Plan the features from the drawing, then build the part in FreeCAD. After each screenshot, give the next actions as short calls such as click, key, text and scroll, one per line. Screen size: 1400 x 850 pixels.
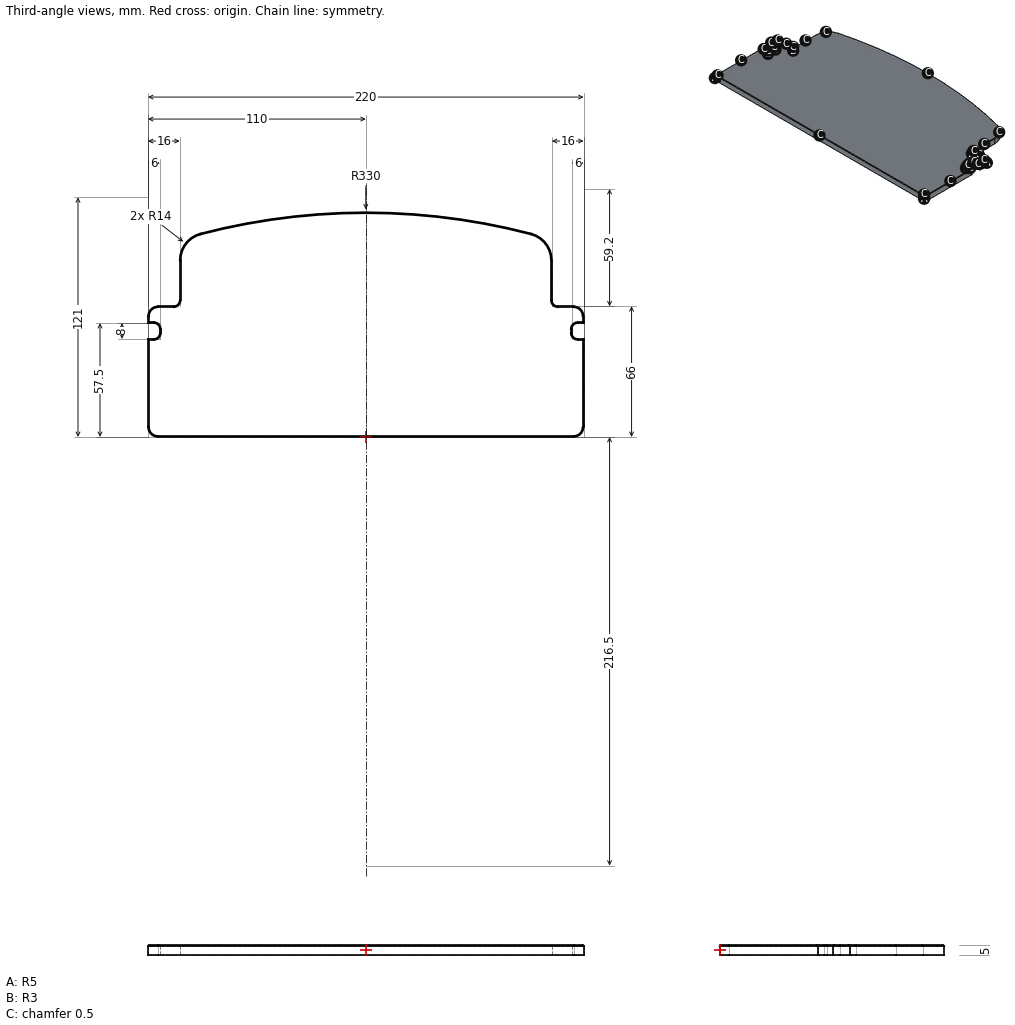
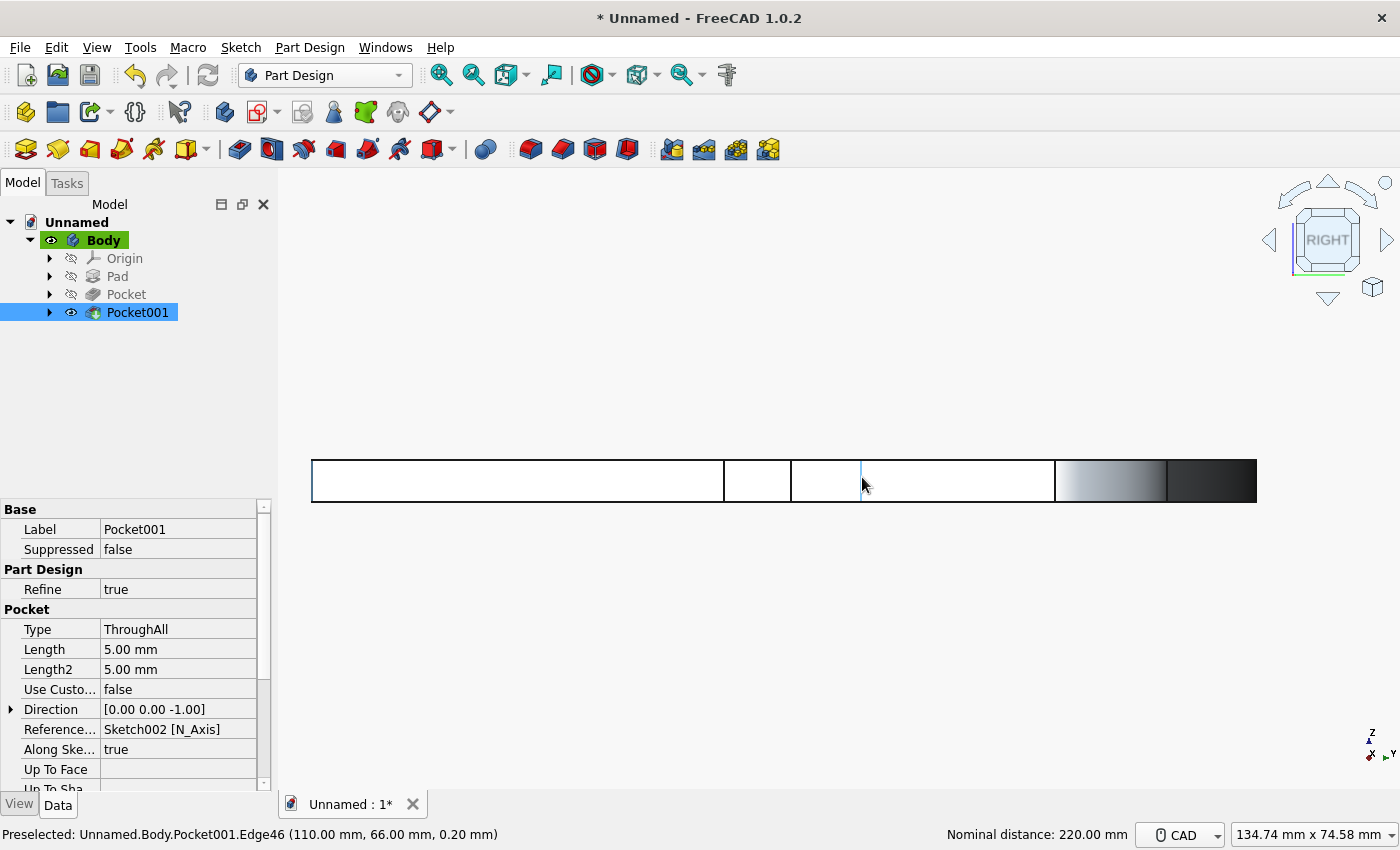
click(861, 480, ctrl)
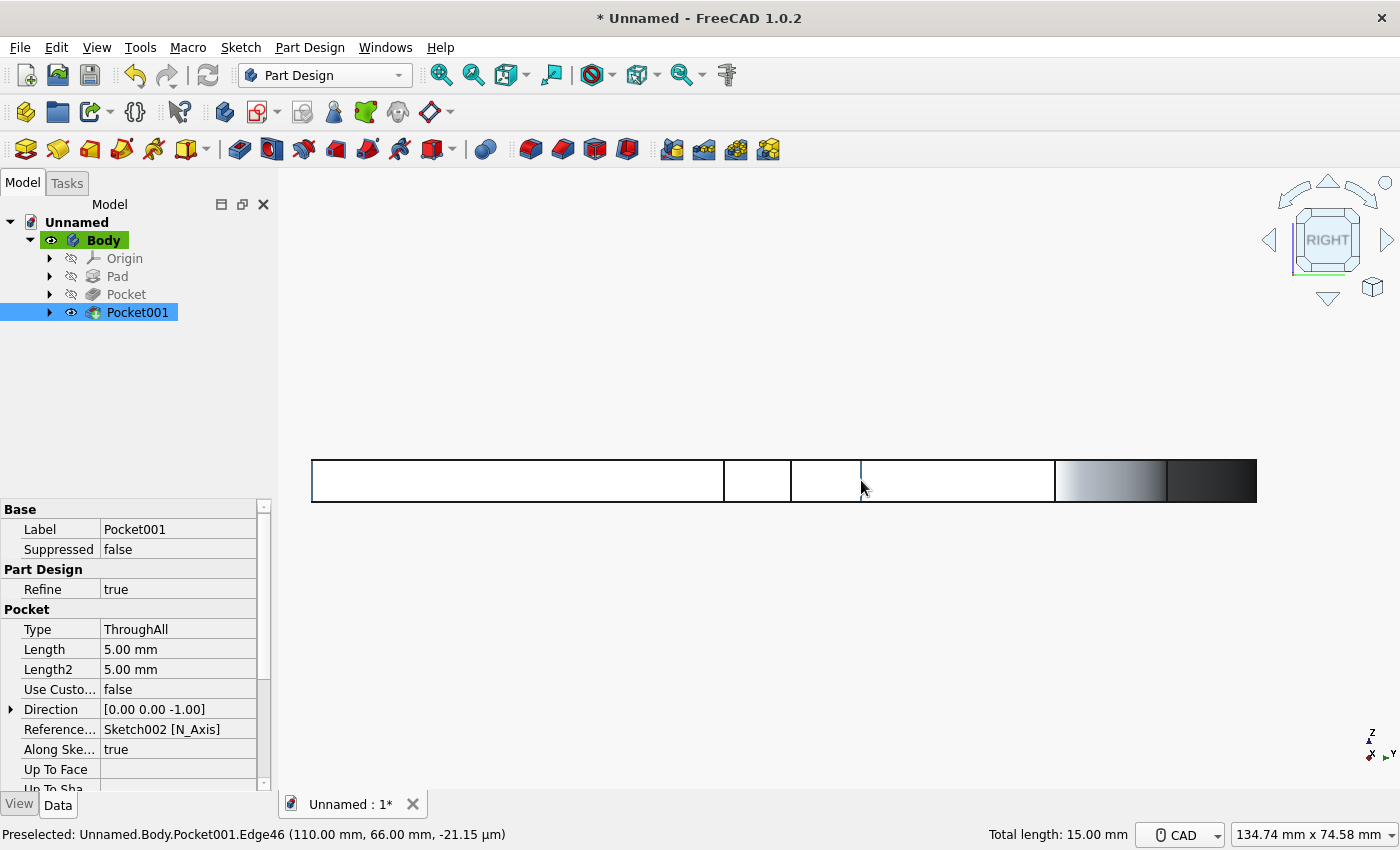
key(v)
key(f)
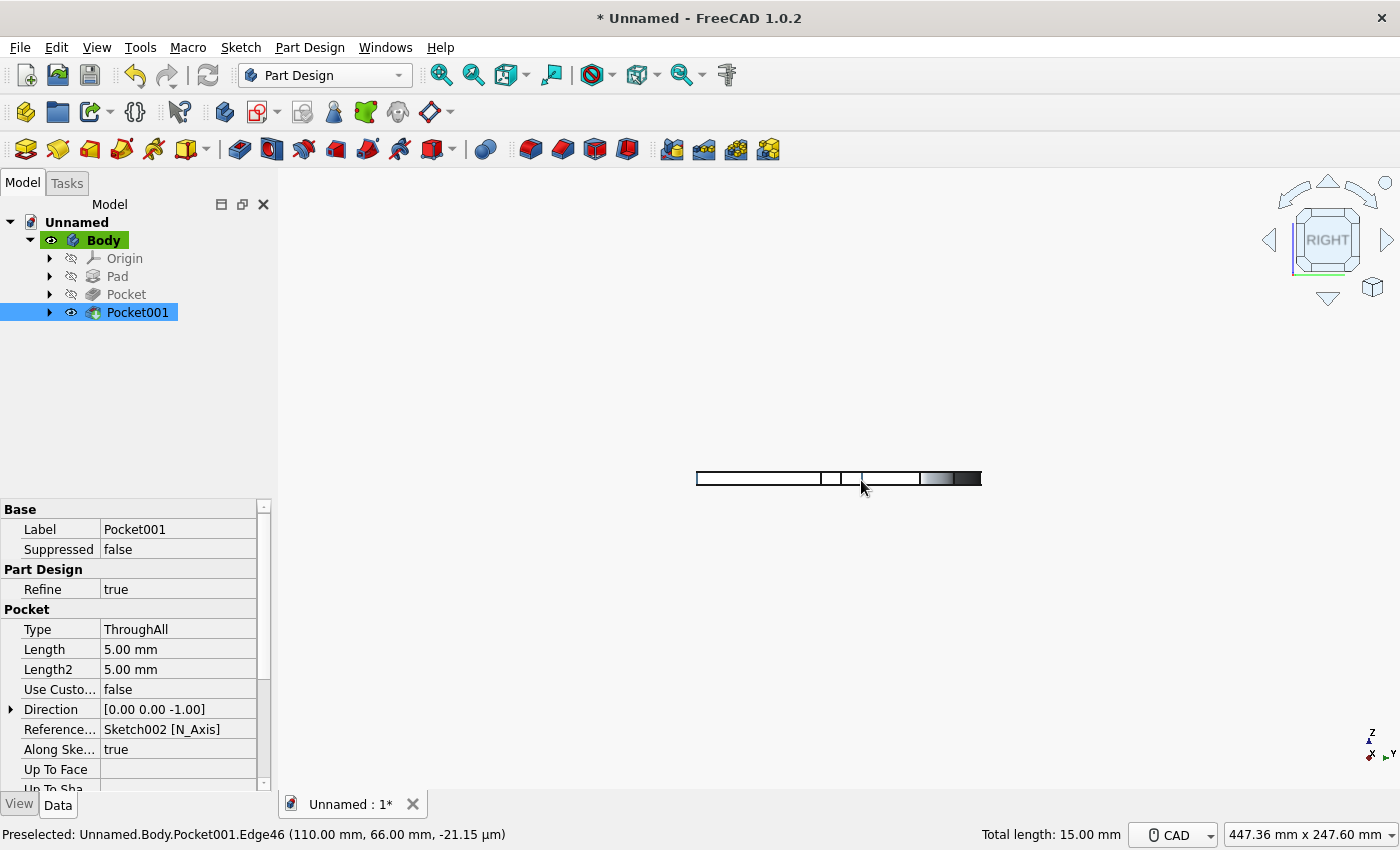
key(5)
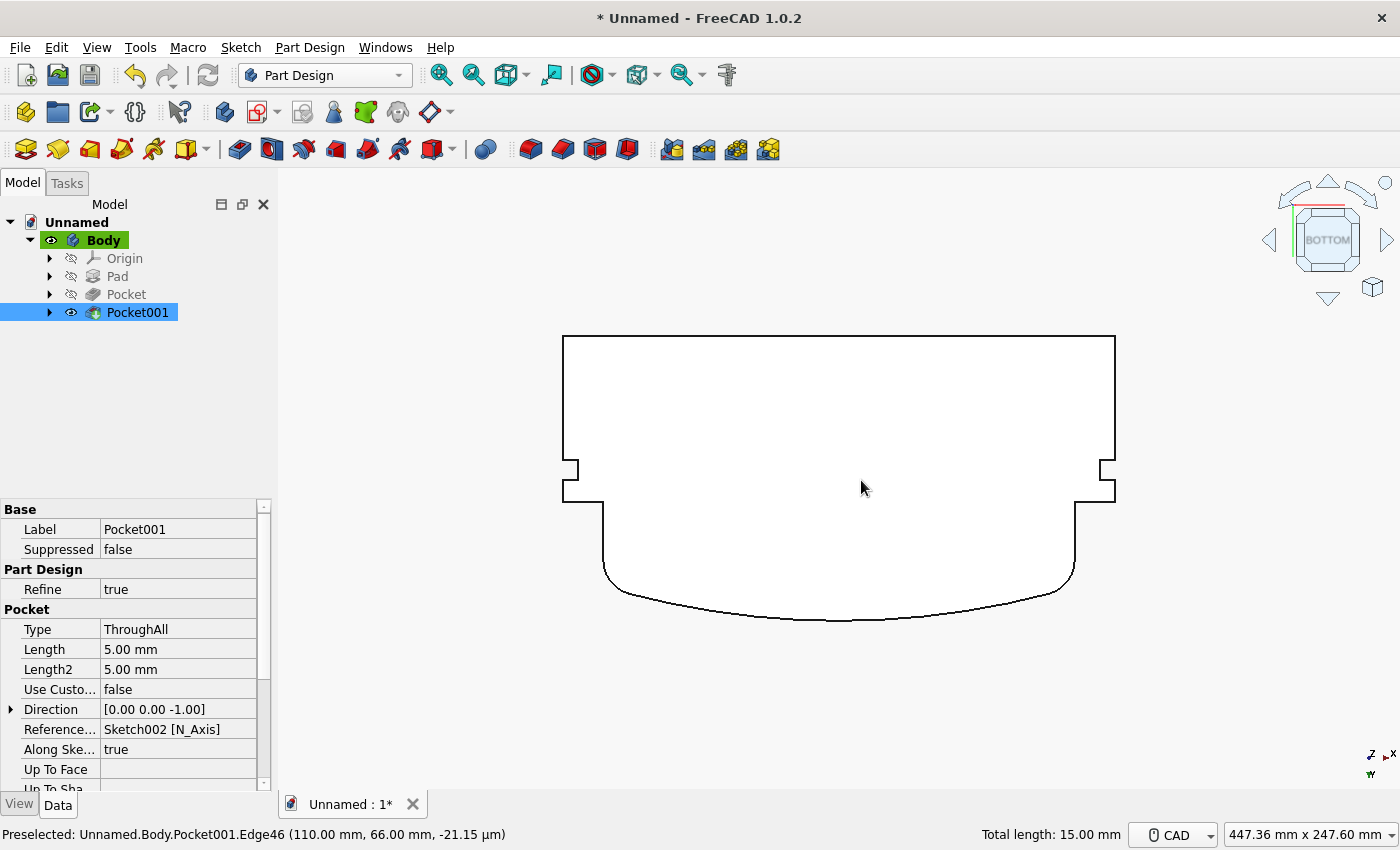
scroll(563, 501, up, 6)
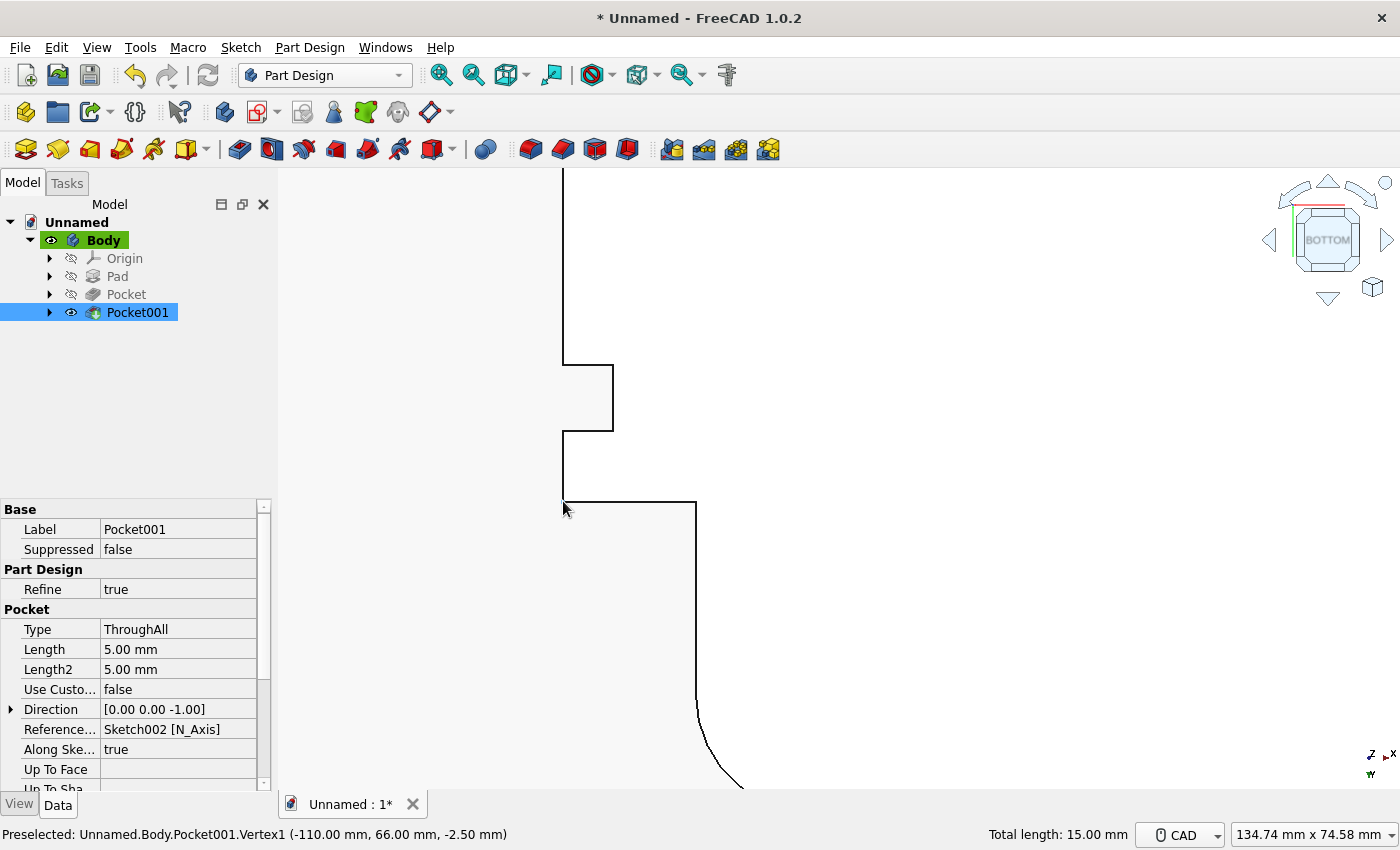
click(442, 76)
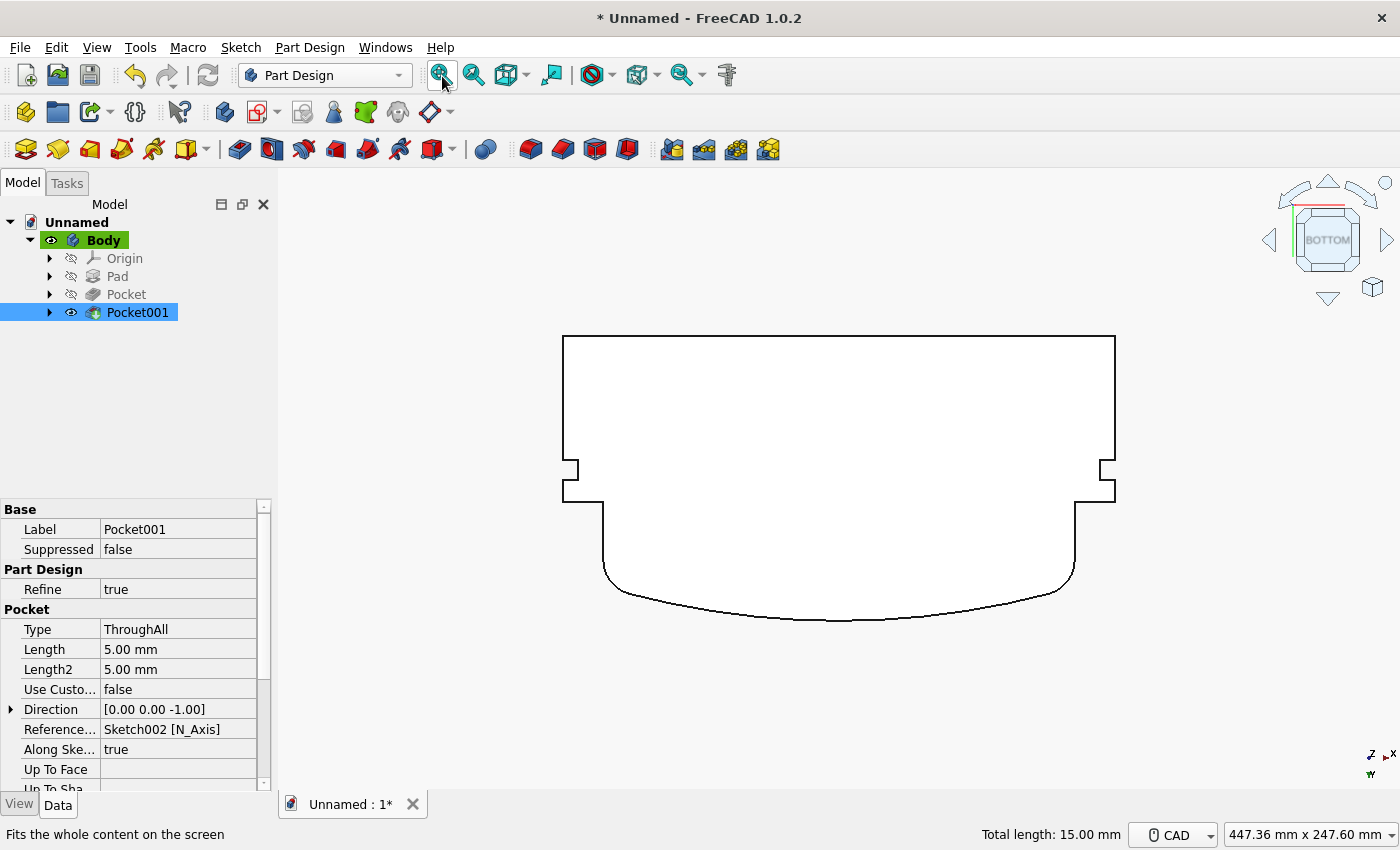
key(4)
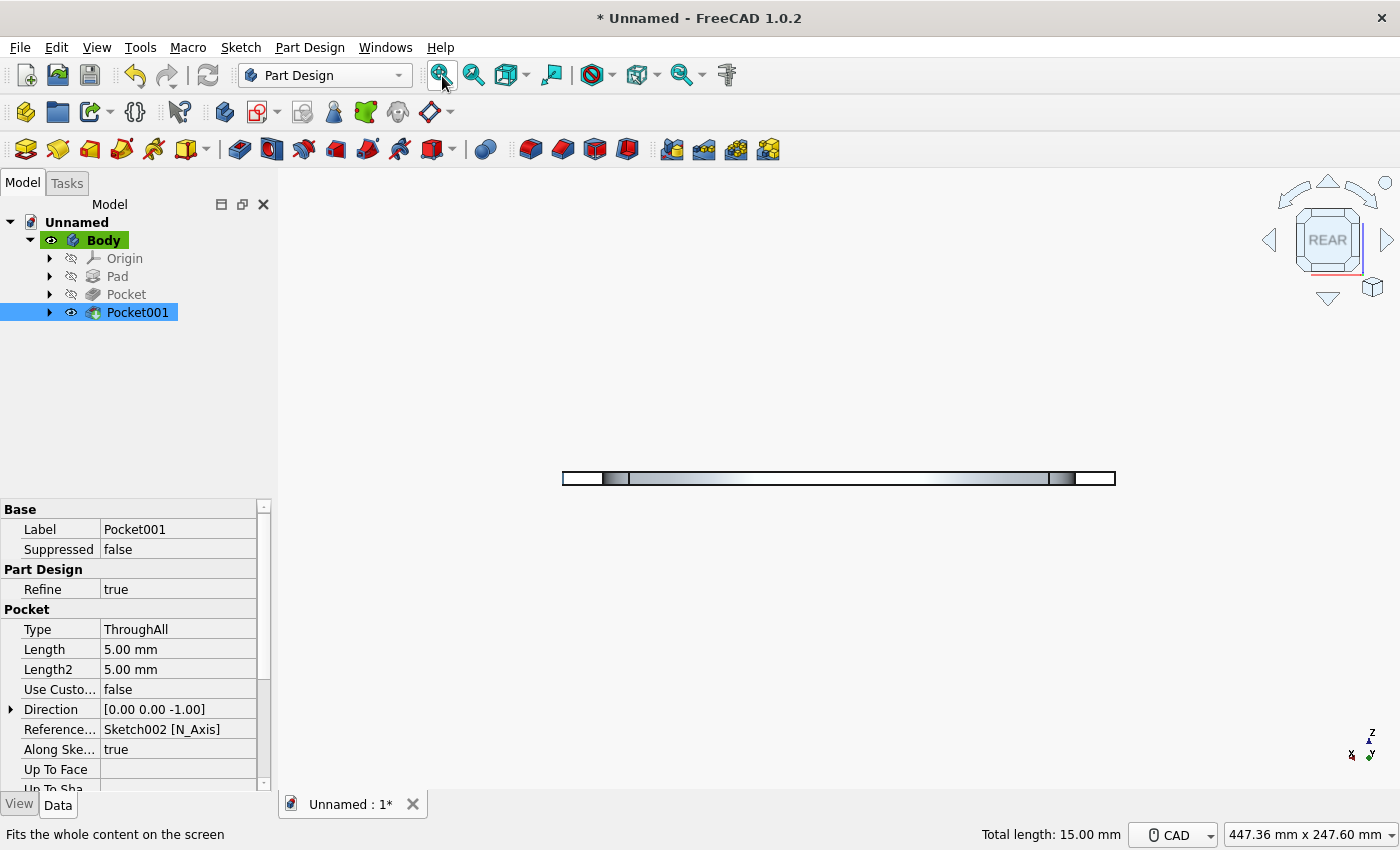
scroll(1115, 477, up, 6)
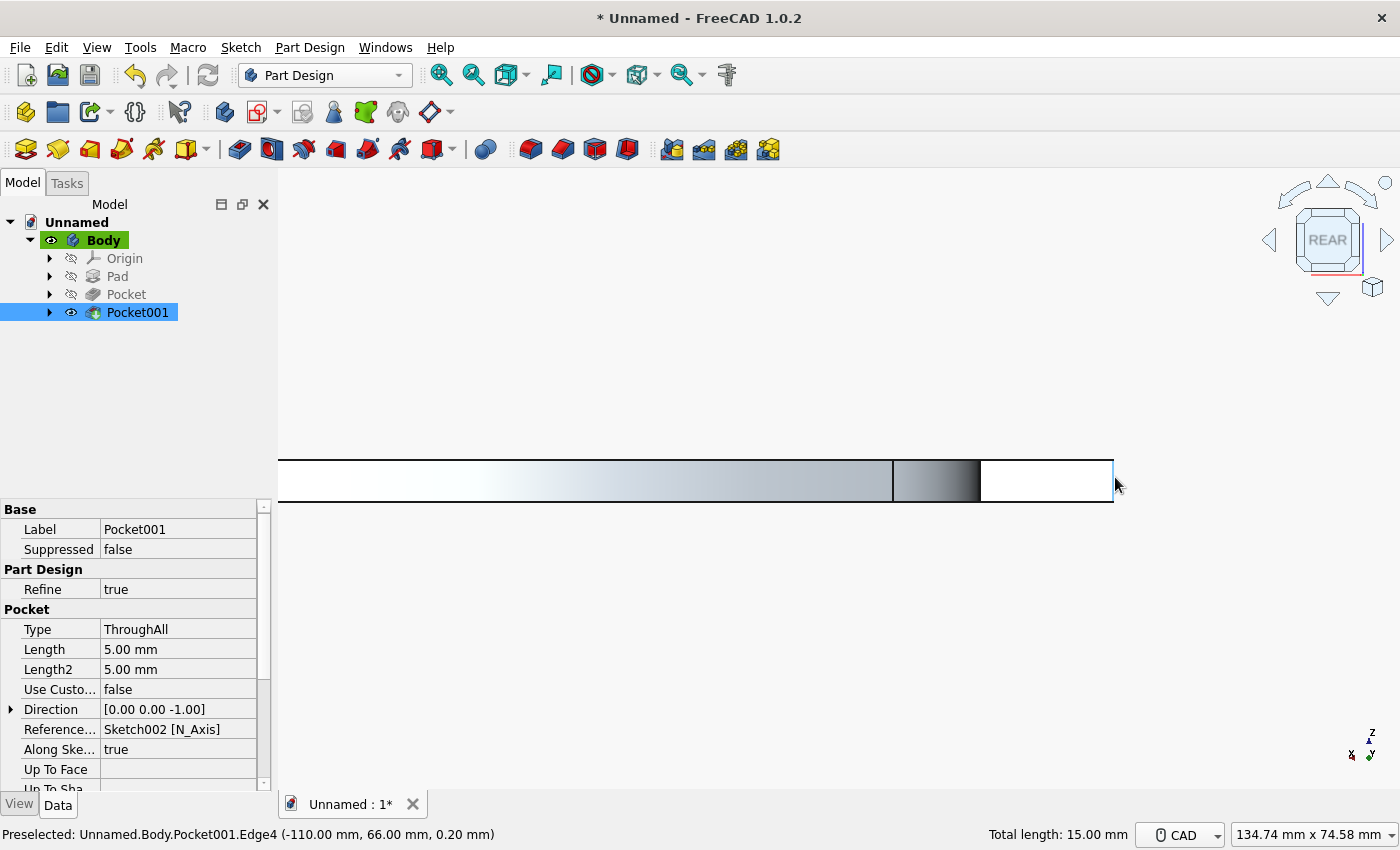
click(1113, 480, ctrl)